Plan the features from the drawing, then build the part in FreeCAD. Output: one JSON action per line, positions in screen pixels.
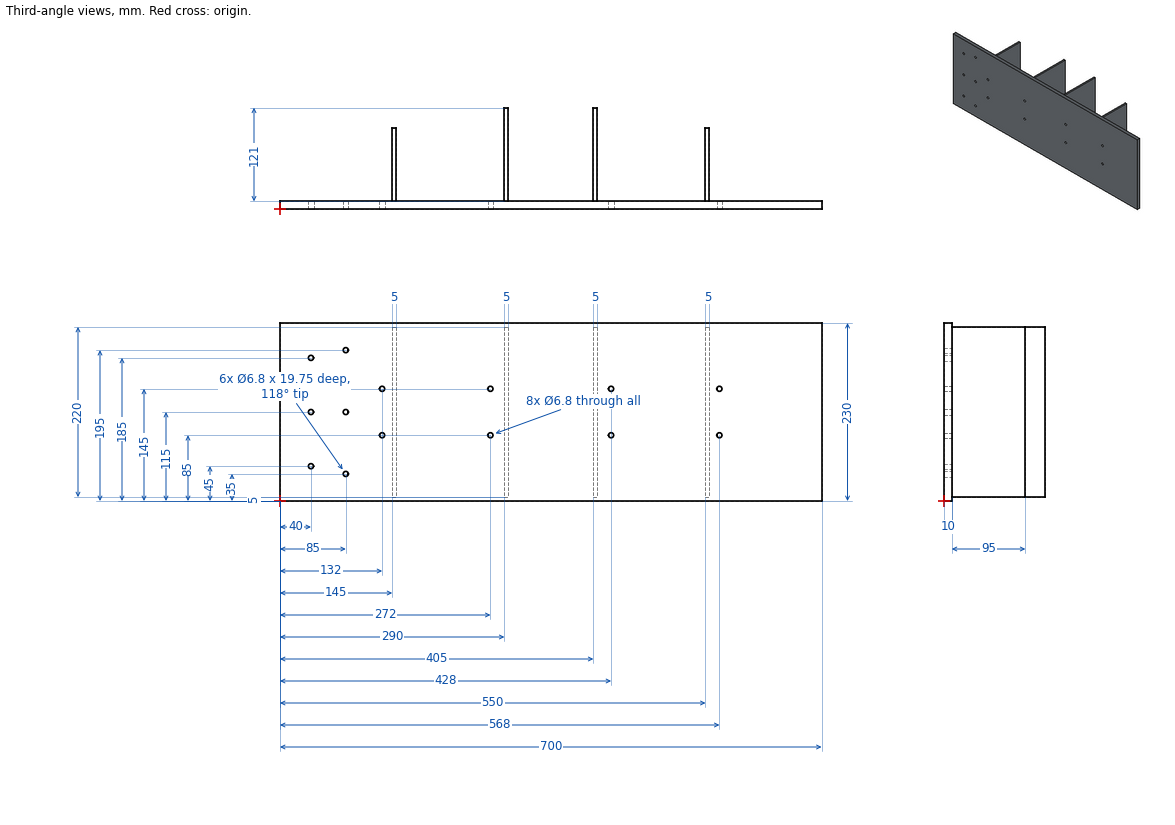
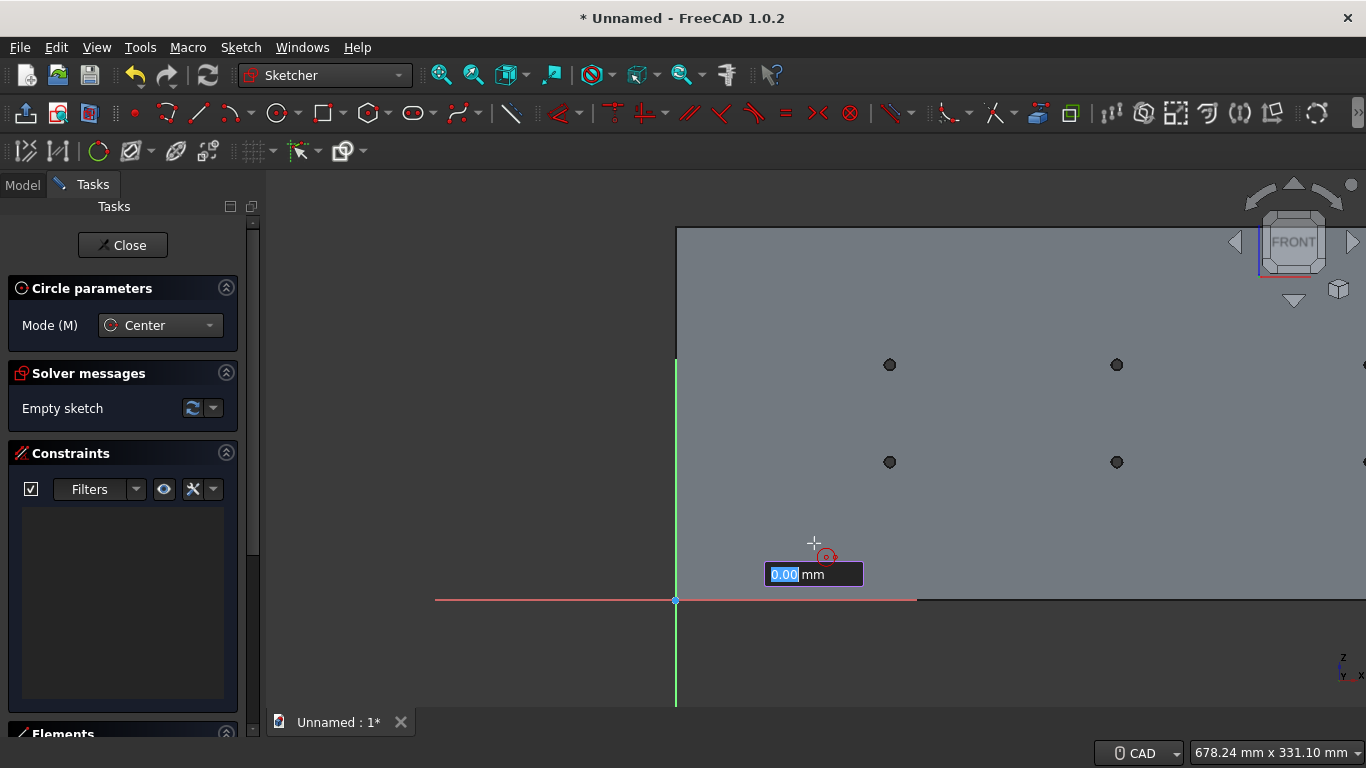
{"action": "scroll", "coordinate": [818, 539], "scroll_direction": "up", "scroll_amount": 6}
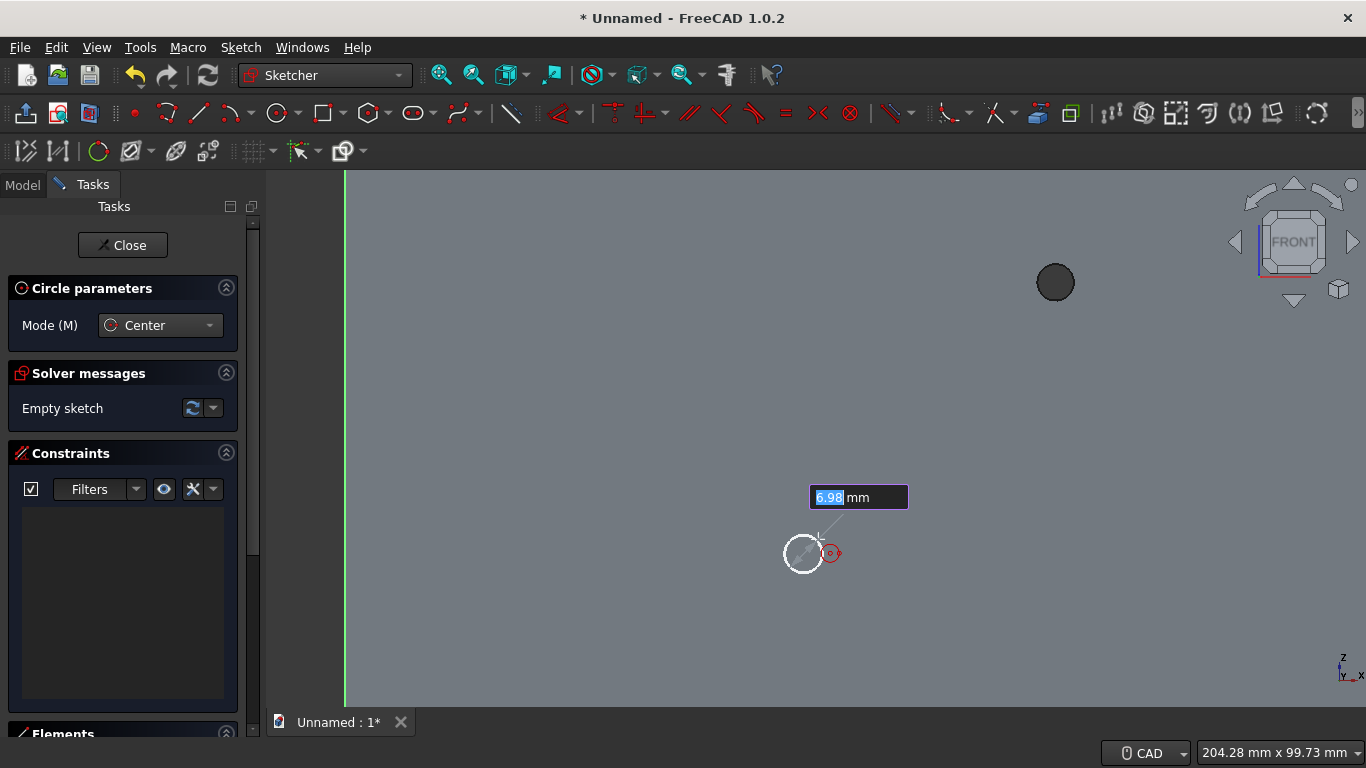
{"action": "left_click", "coordinate": [816, 539]}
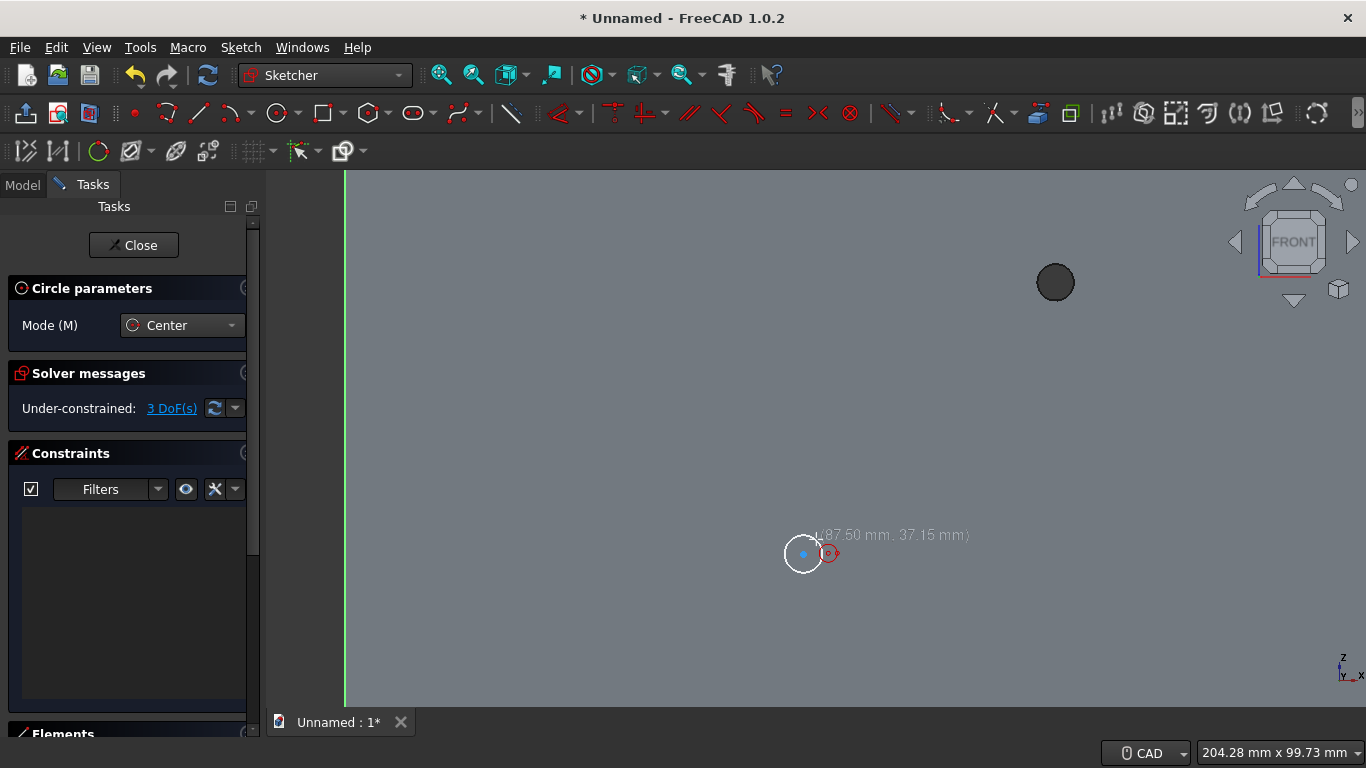
{"action": "scroll", "coordinate": [560, 498], "scroll_direction": "up", "scroll_amount": 2}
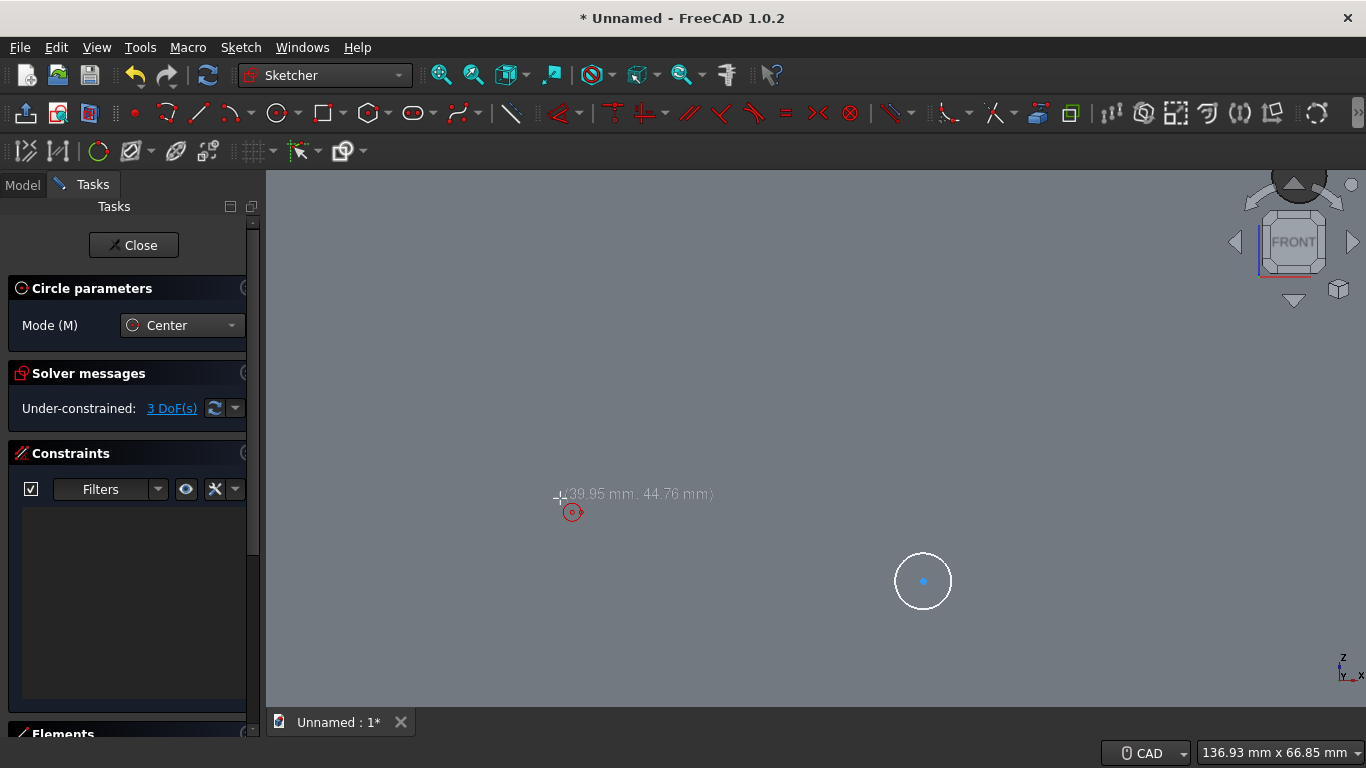
{"action": "scroll", "coordinate": [786, 534], "scroll_direction": "down", "scroll_amount": 8}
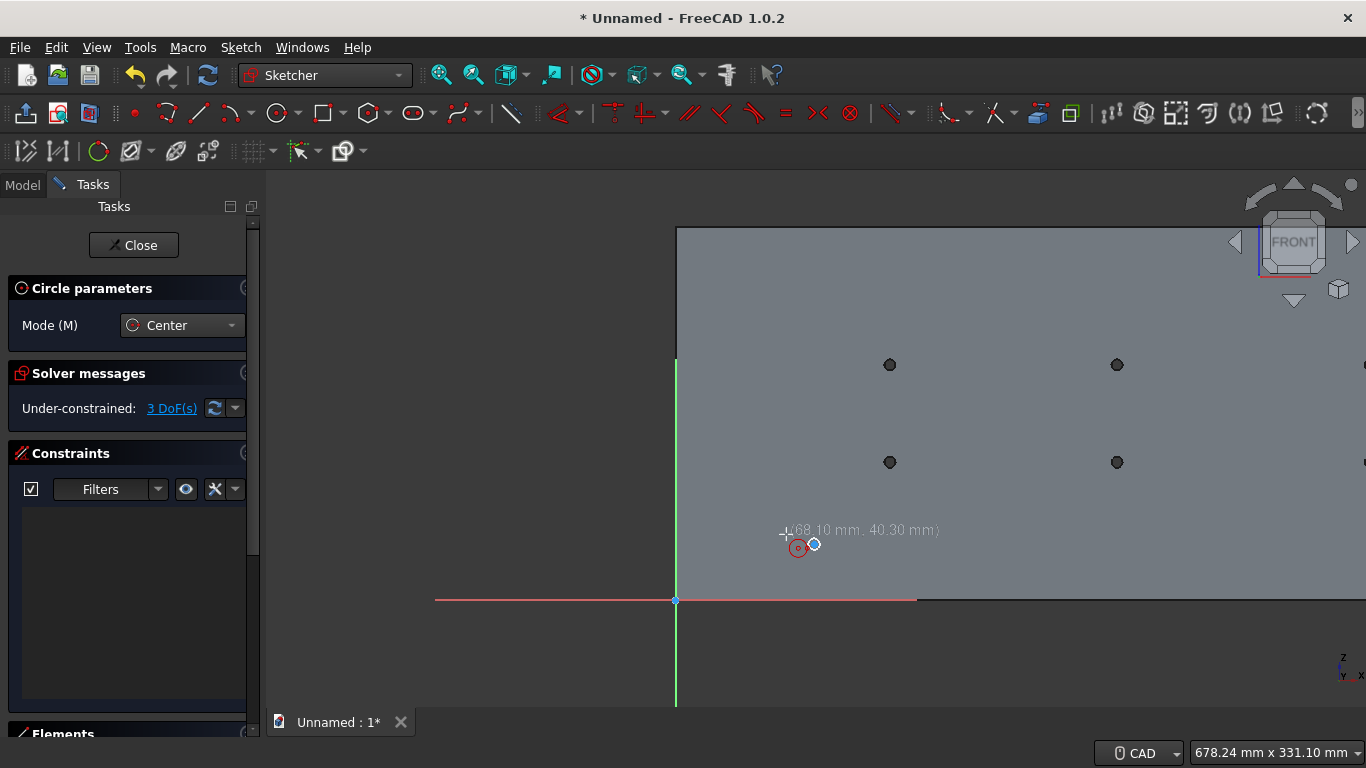
{"action": "left_click", "coordinate": [741, 527]}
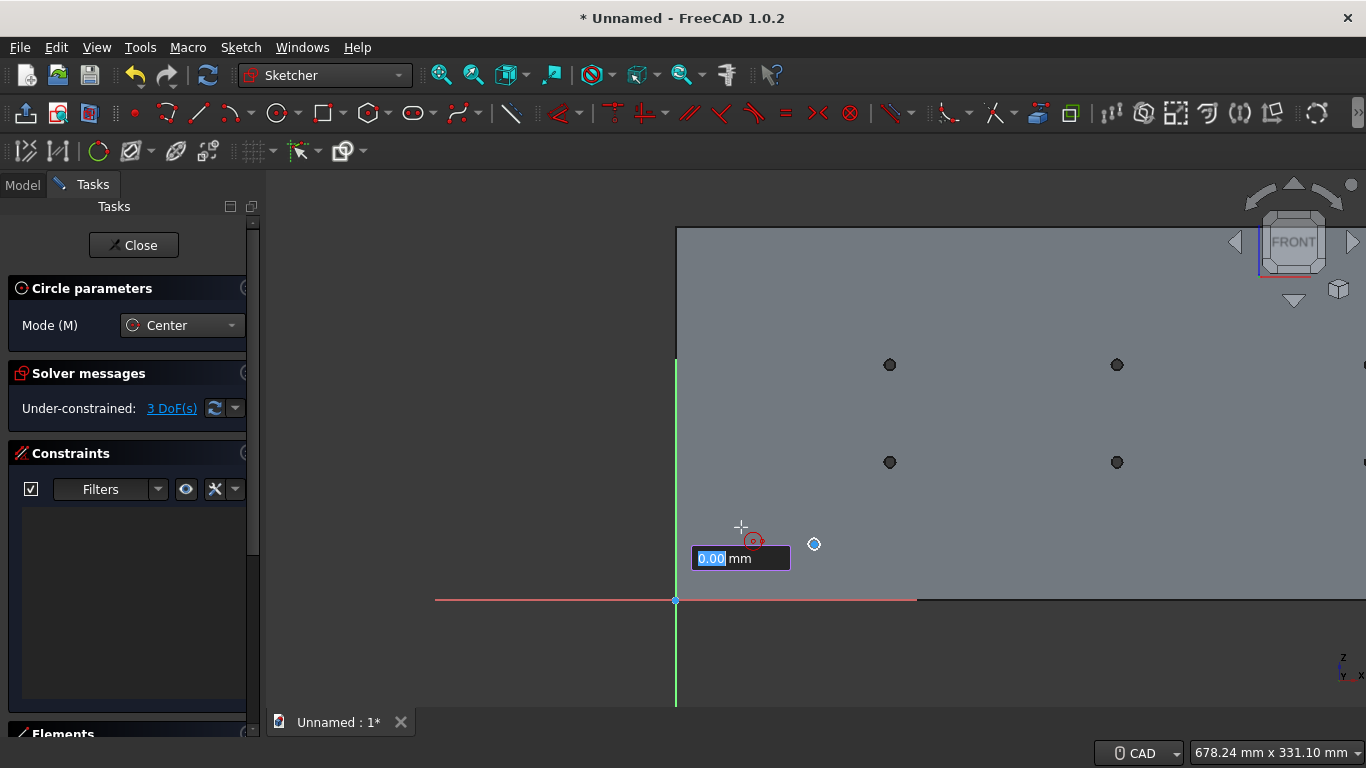
{"action": "scroll", "coordinate": [745, 523], "scroll_direction": "up", "scroll_amount": 6}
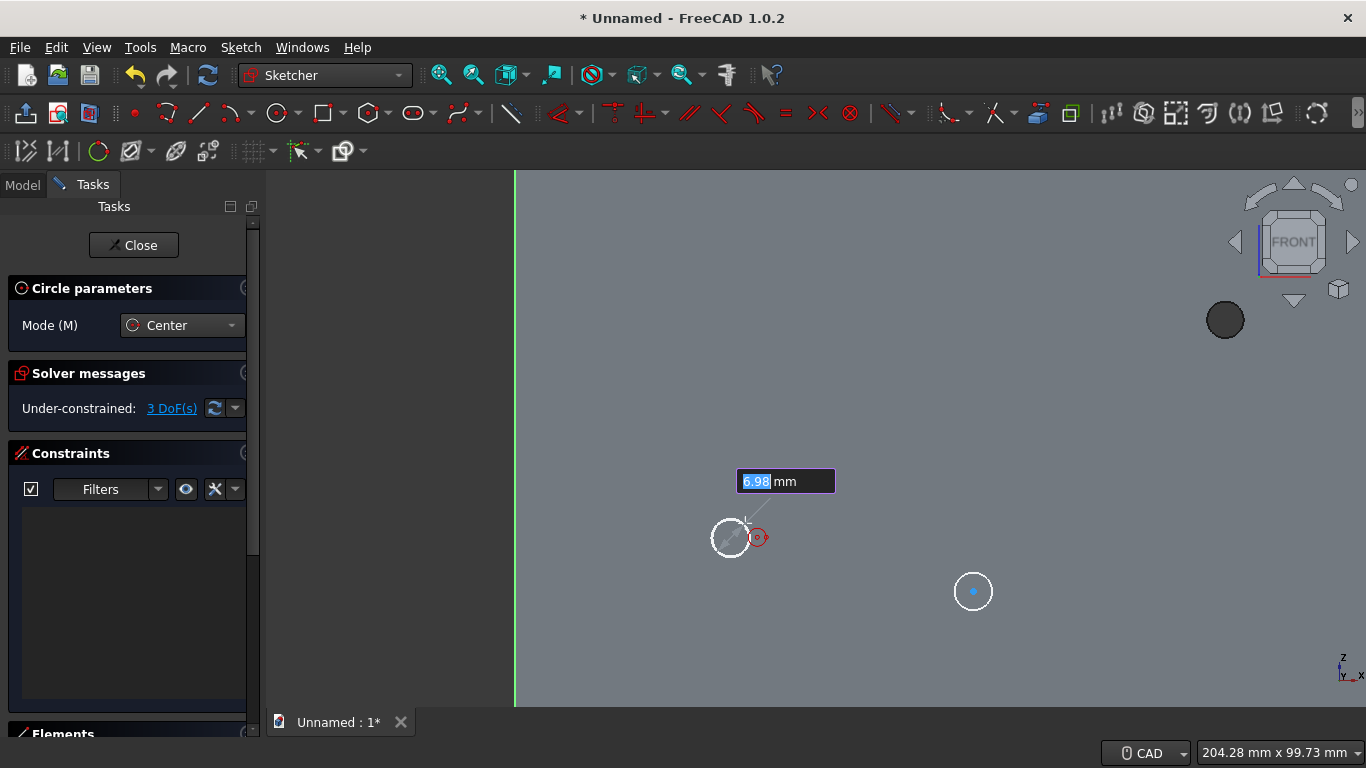
{"action": "left_click", "coordinate": [743, 522]}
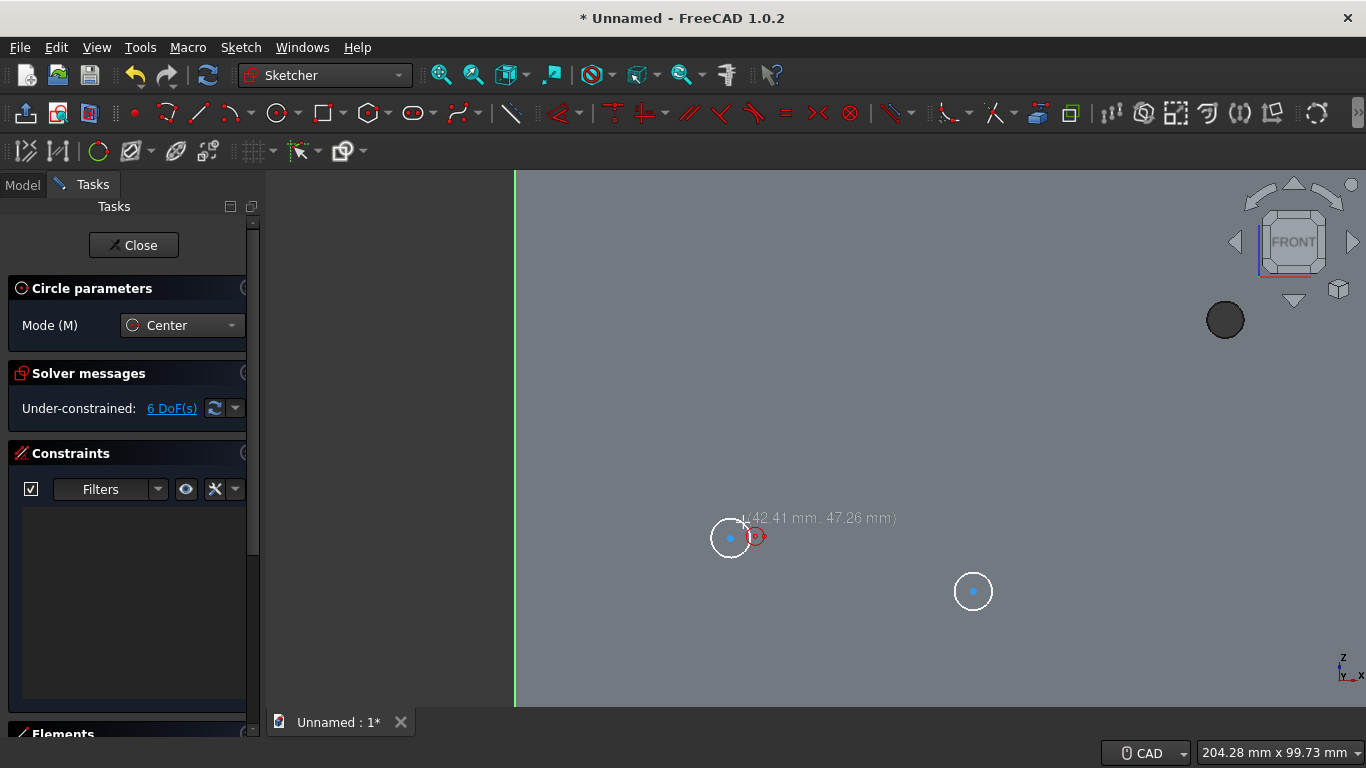
{"action": "scroll", "coordinate": [745, 523], "scroll_direction": "down", "scroll_amount": 6}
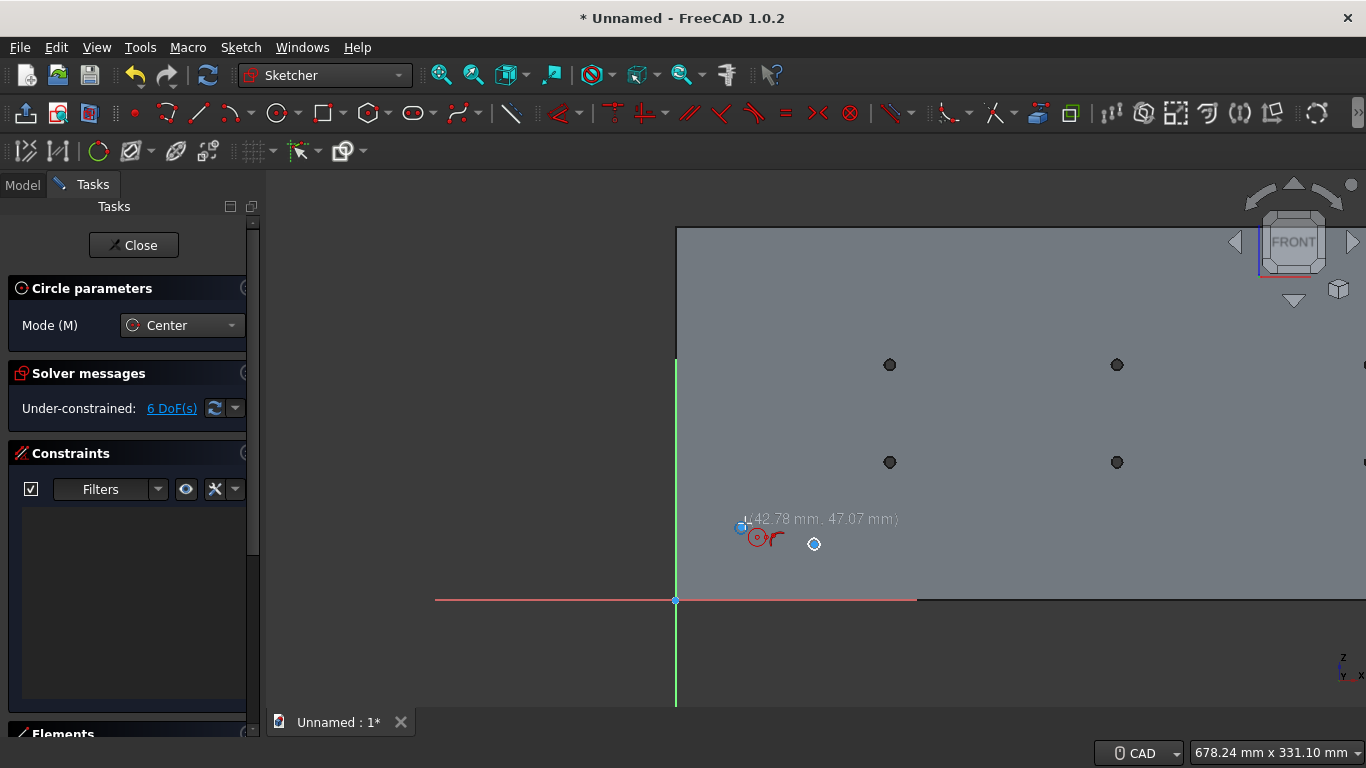
{"action": "scroll", "coordinate": [741, 300], "scroll_direction": "up", "scroll_amount": 8}